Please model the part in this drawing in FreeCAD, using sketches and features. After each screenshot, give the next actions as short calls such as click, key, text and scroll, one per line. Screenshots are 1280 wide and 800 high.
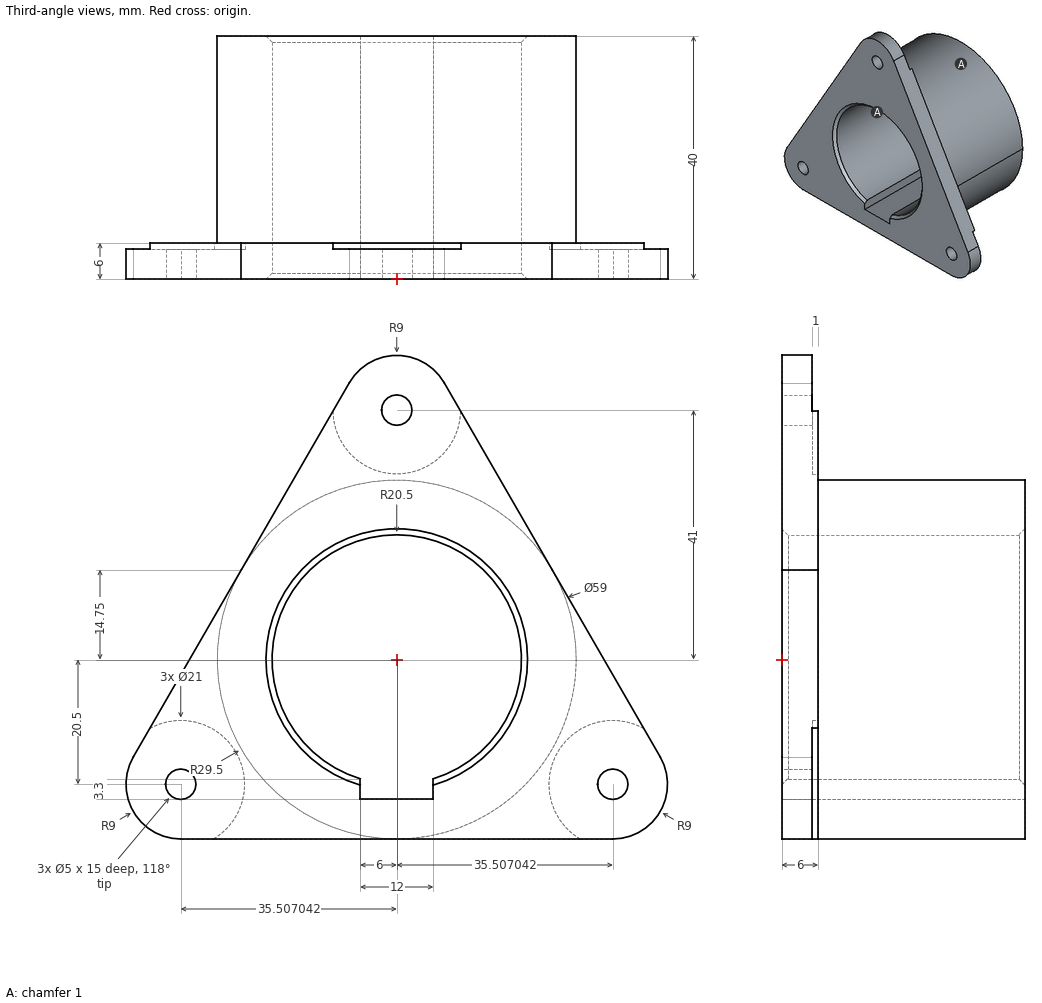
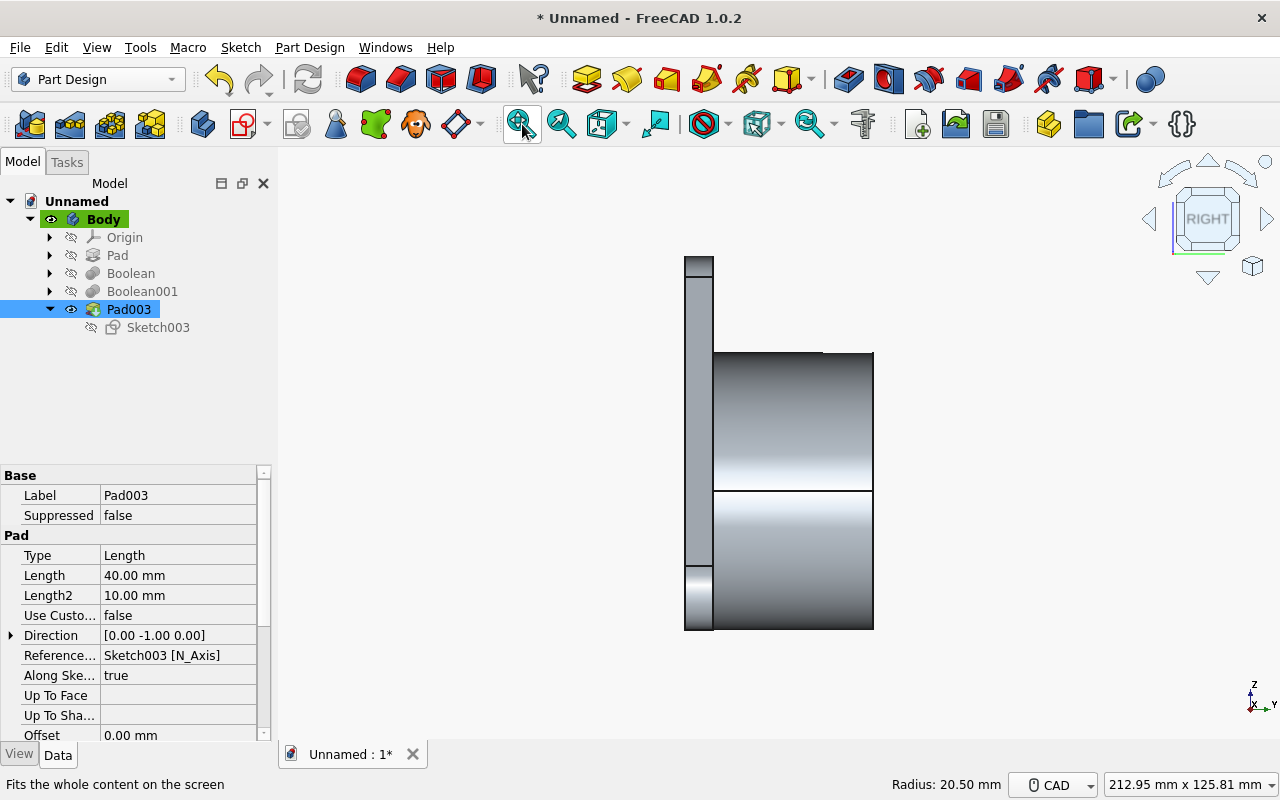
key(5)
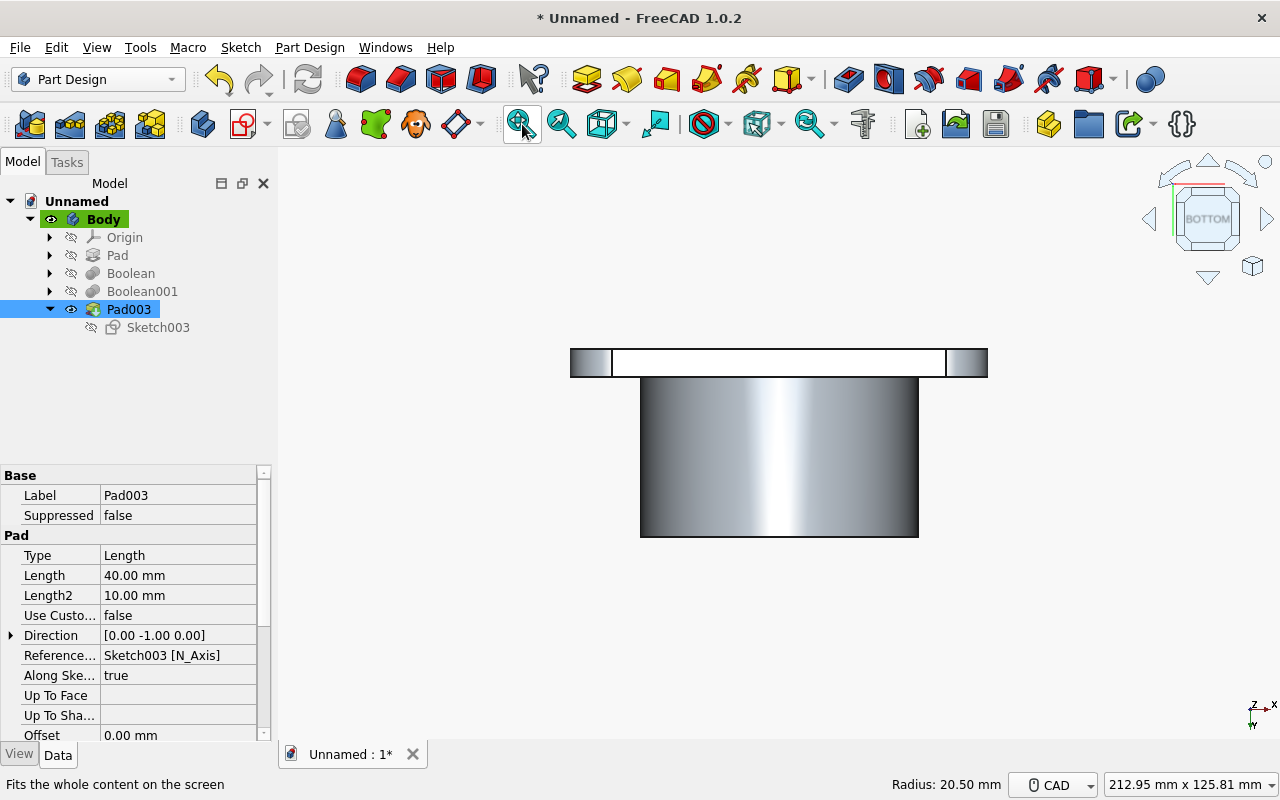
click(522, 124)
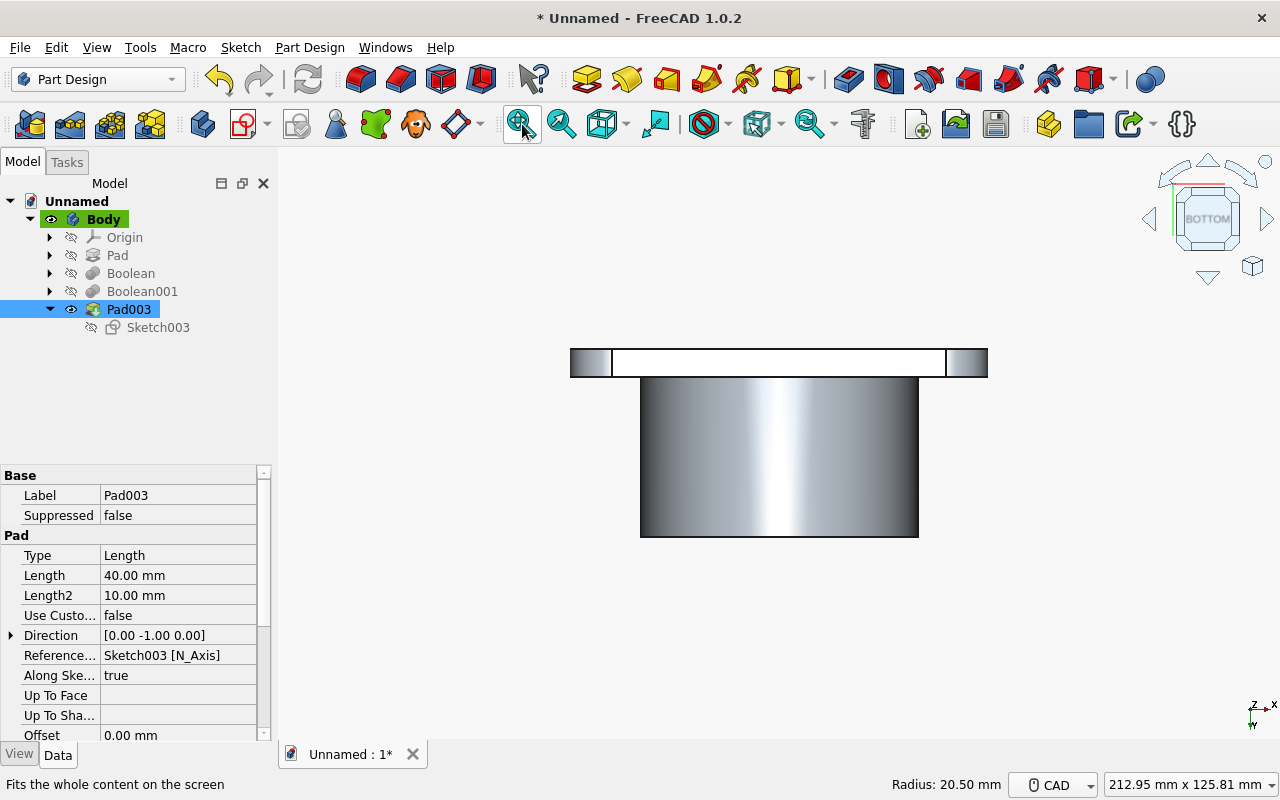
key(4)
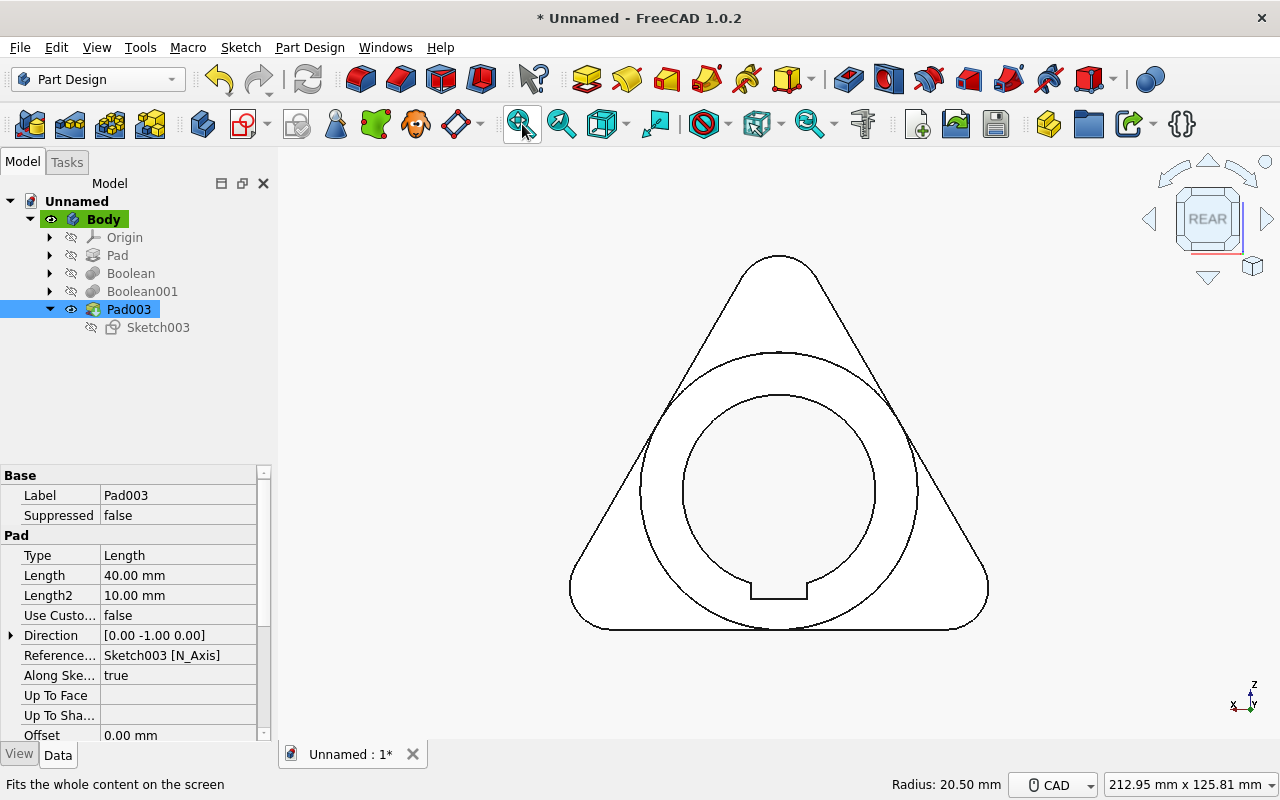
click(779, 394, ctrl)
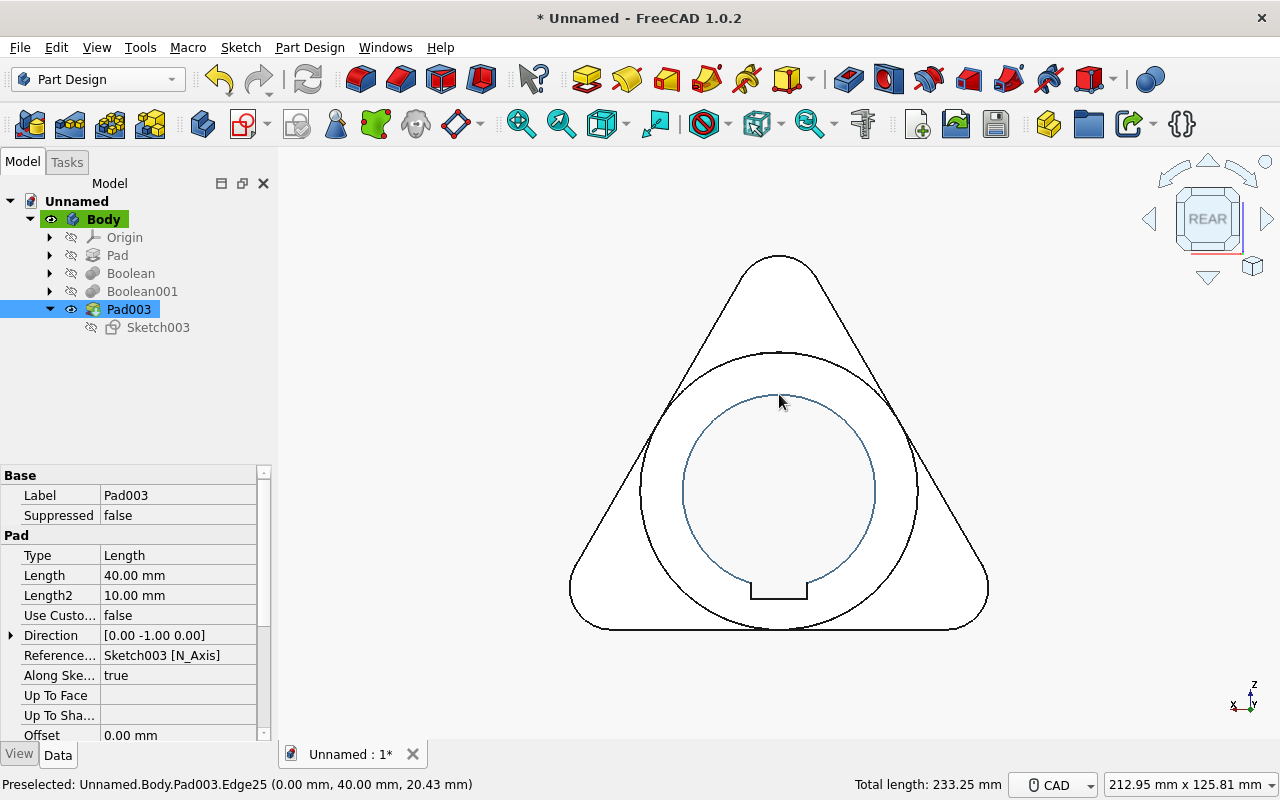
click(402, 80)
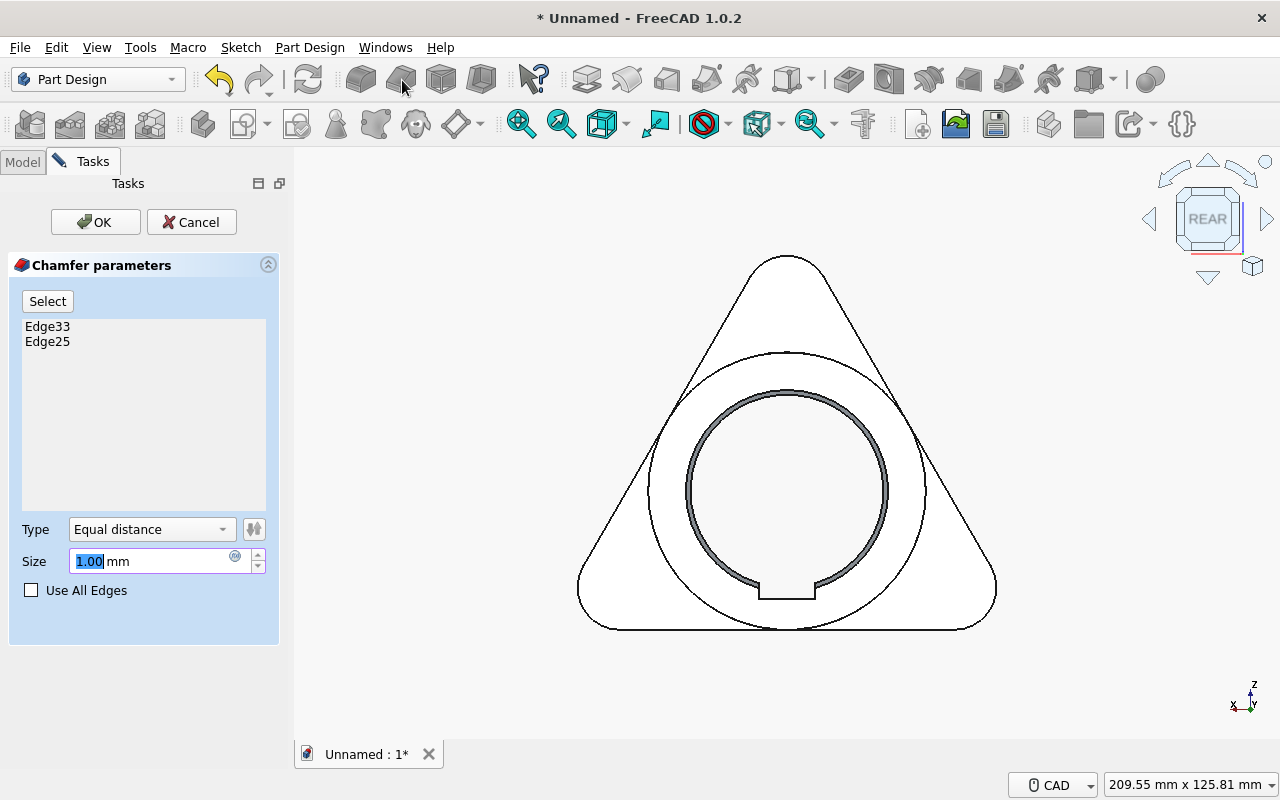
text(1)
key(Tab)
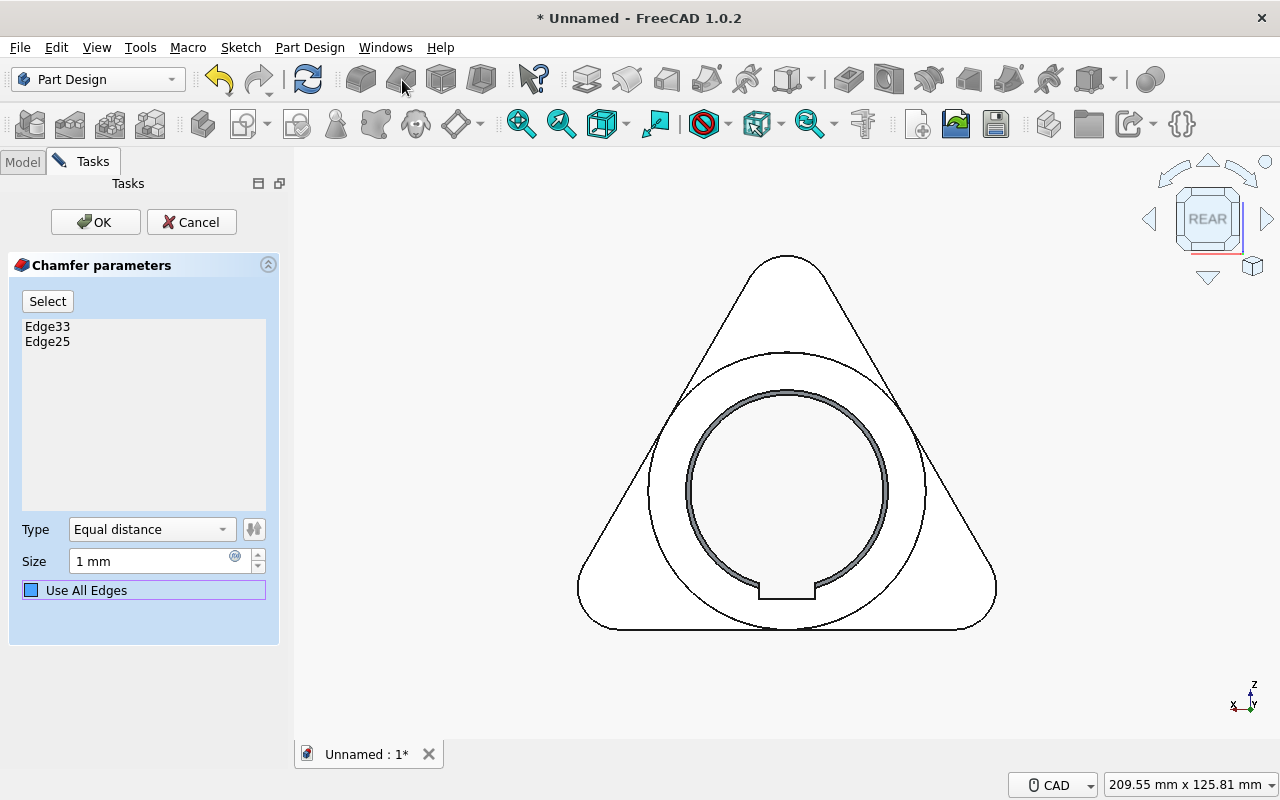
click(96, 222)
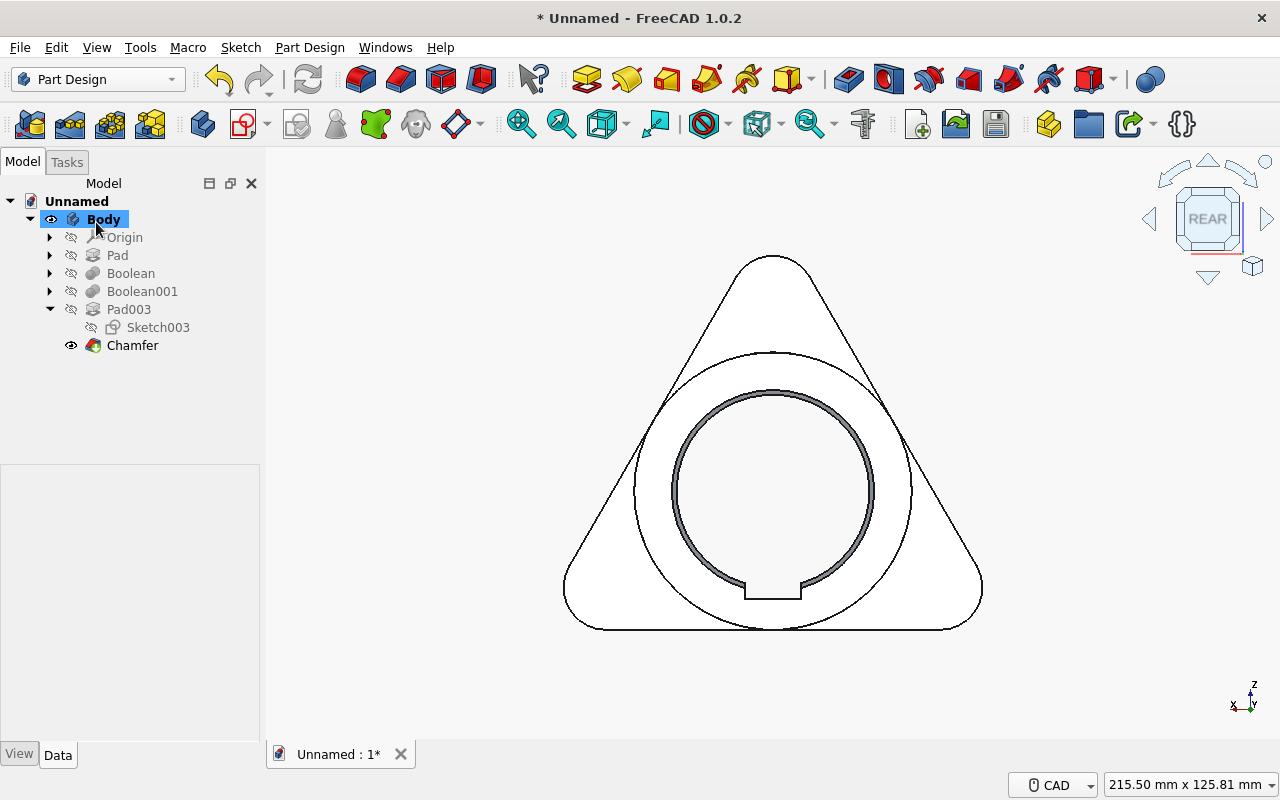
click(773, 314)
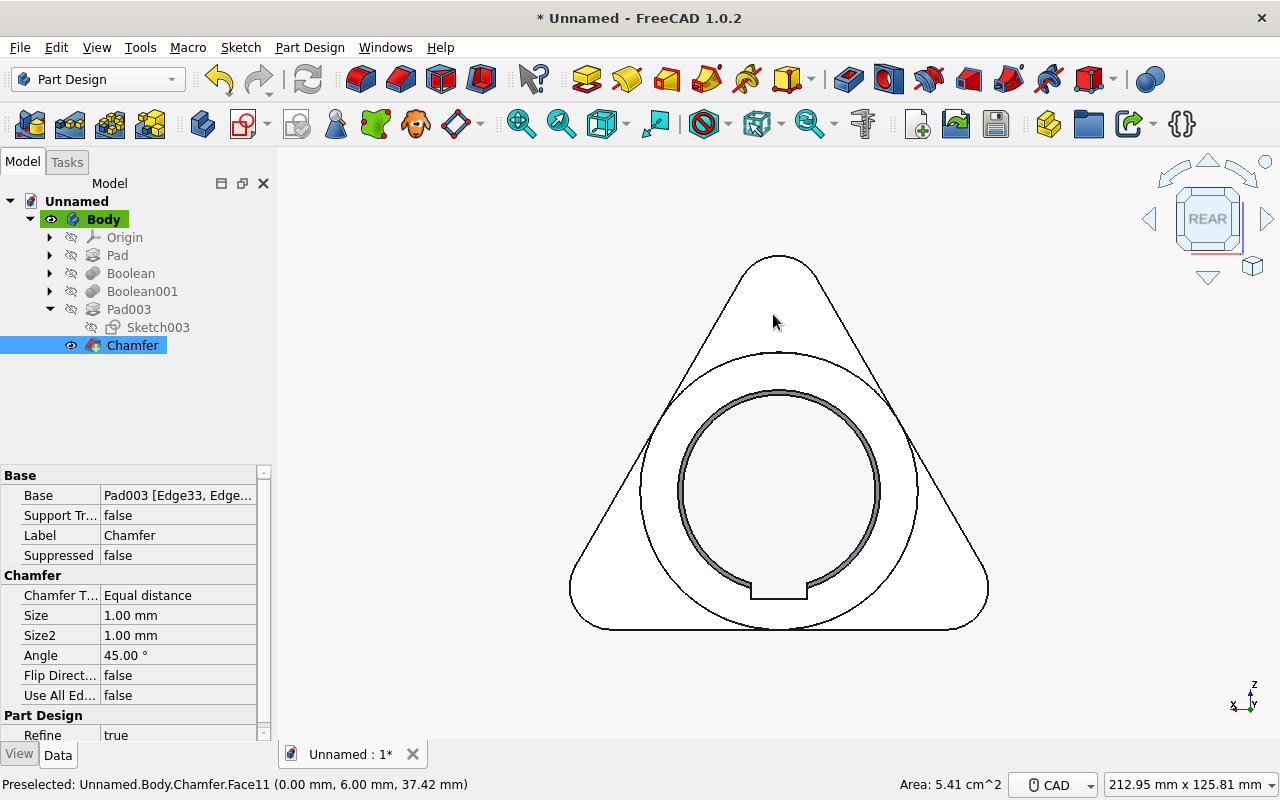
click(244, 124)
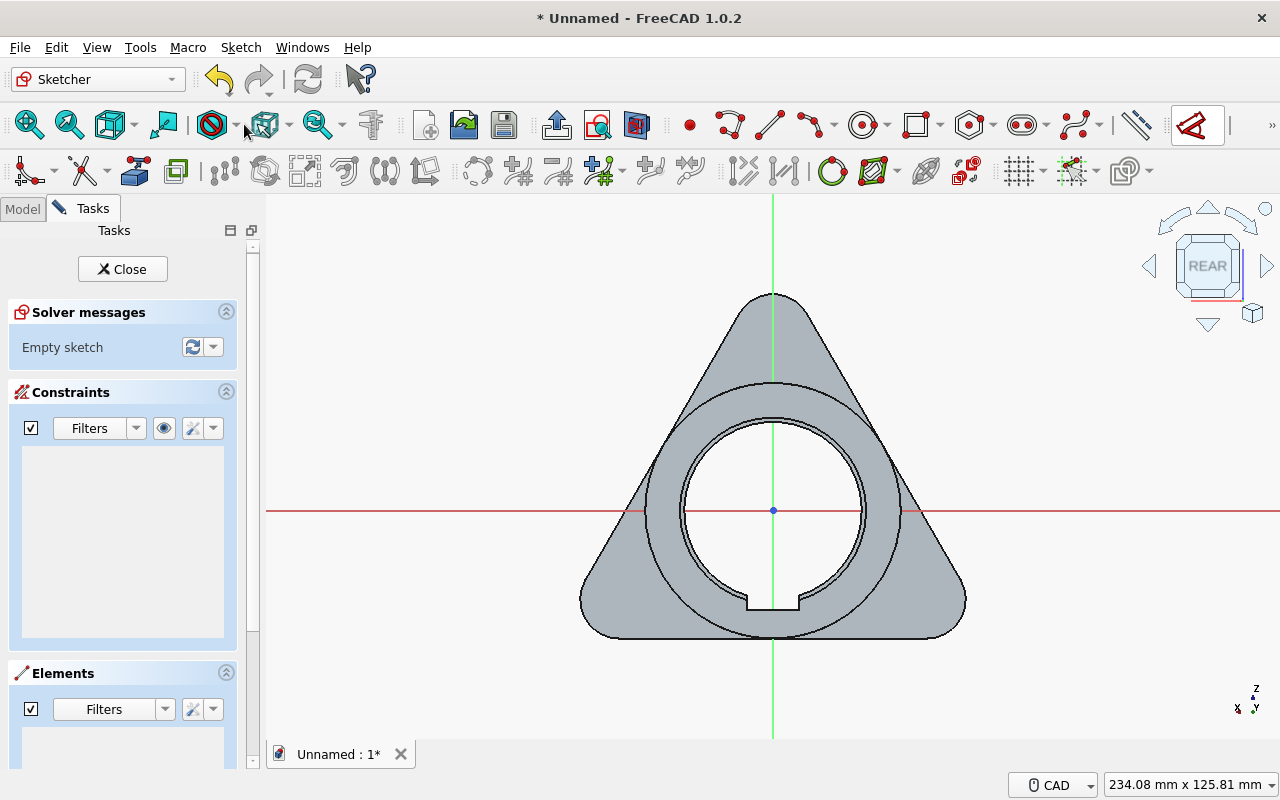
click(864, 126)